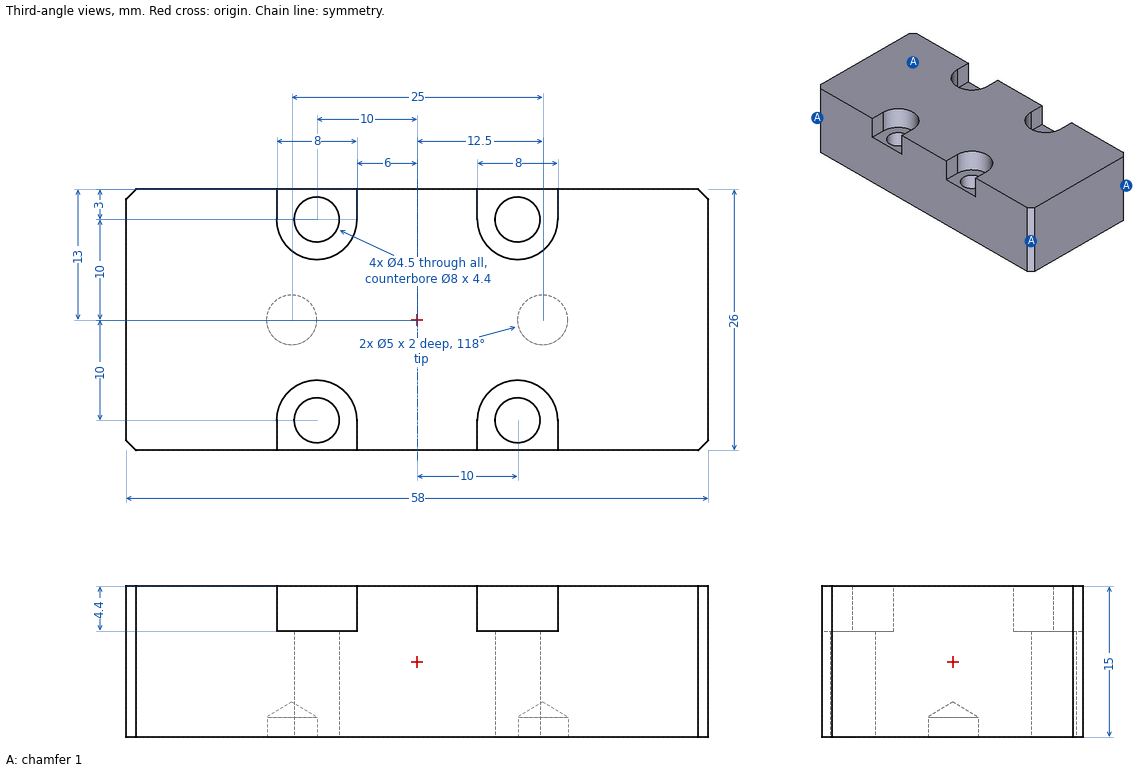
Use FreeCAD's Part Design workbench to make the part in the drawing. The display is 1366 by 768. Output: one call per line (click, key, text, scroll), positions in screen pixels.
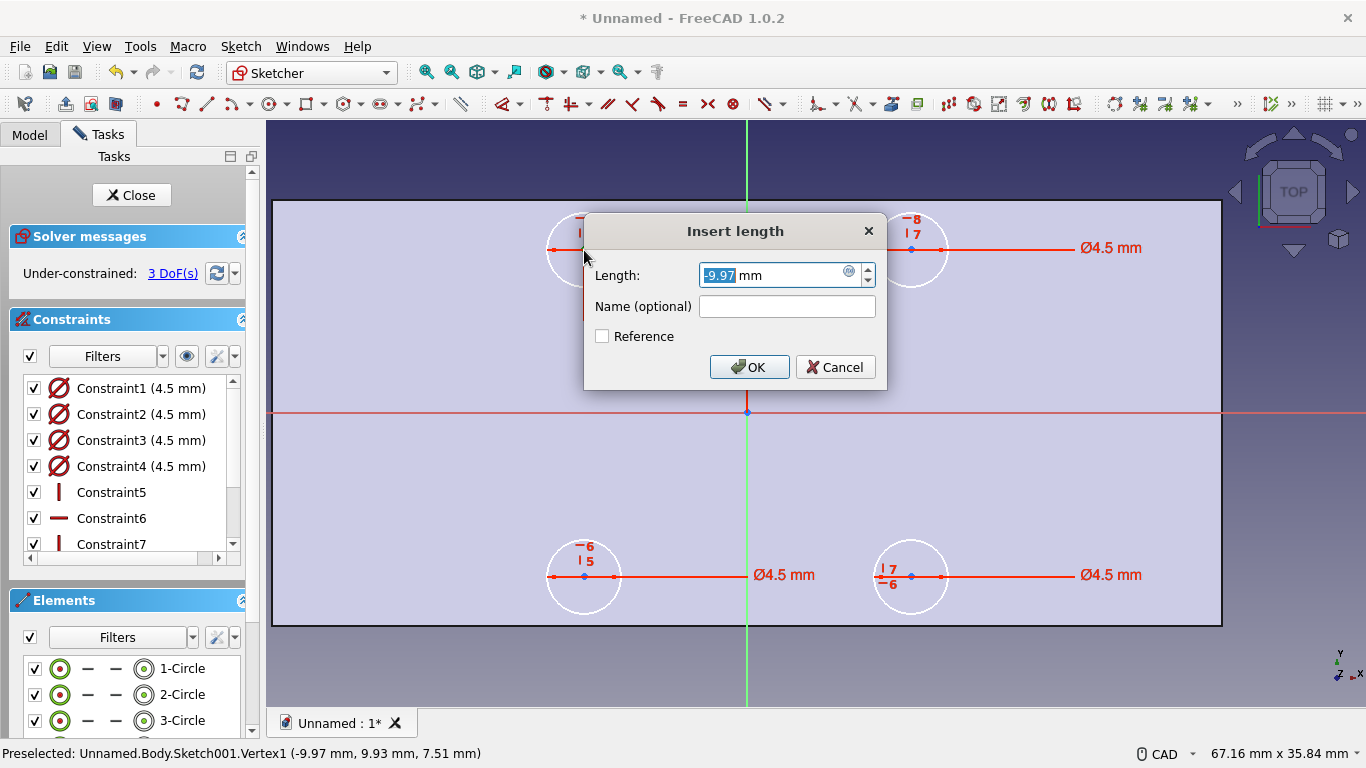
text(-10)
key(Return)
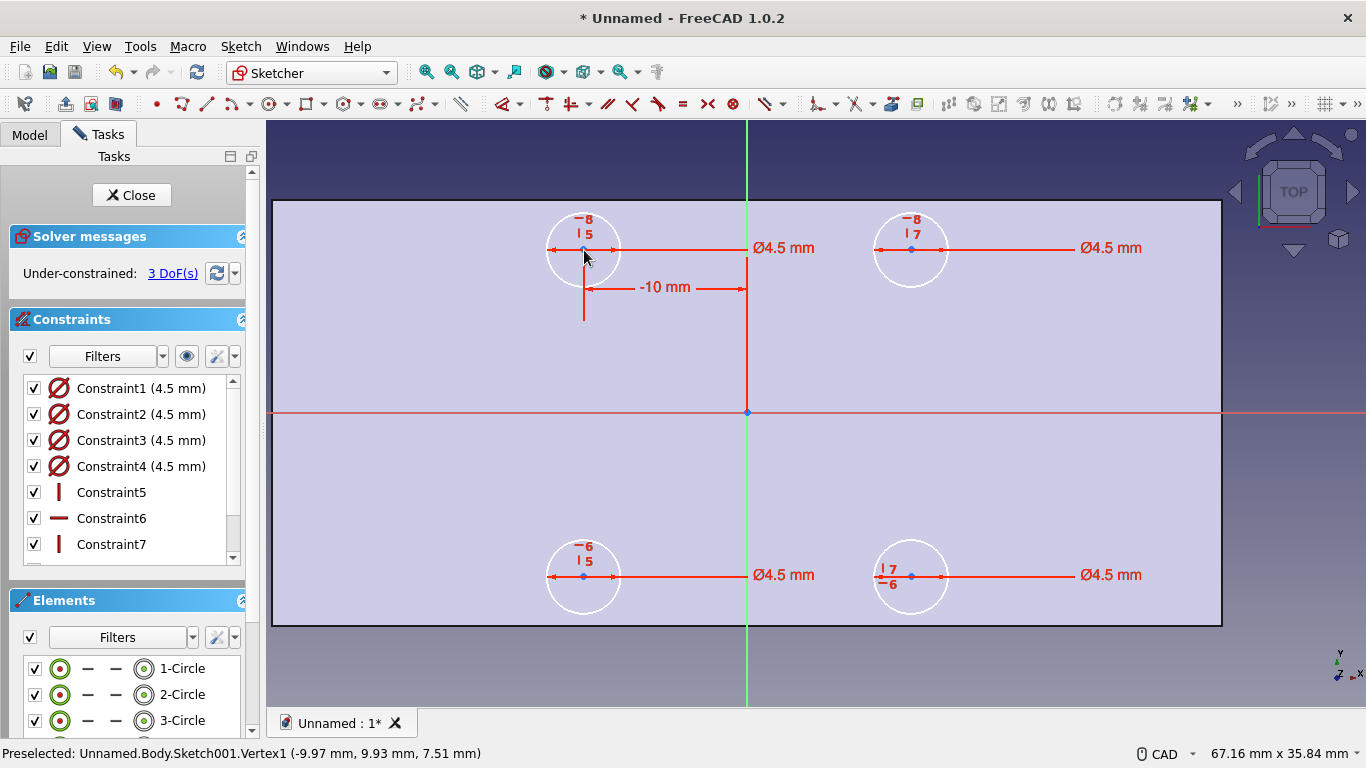
click(584, 250)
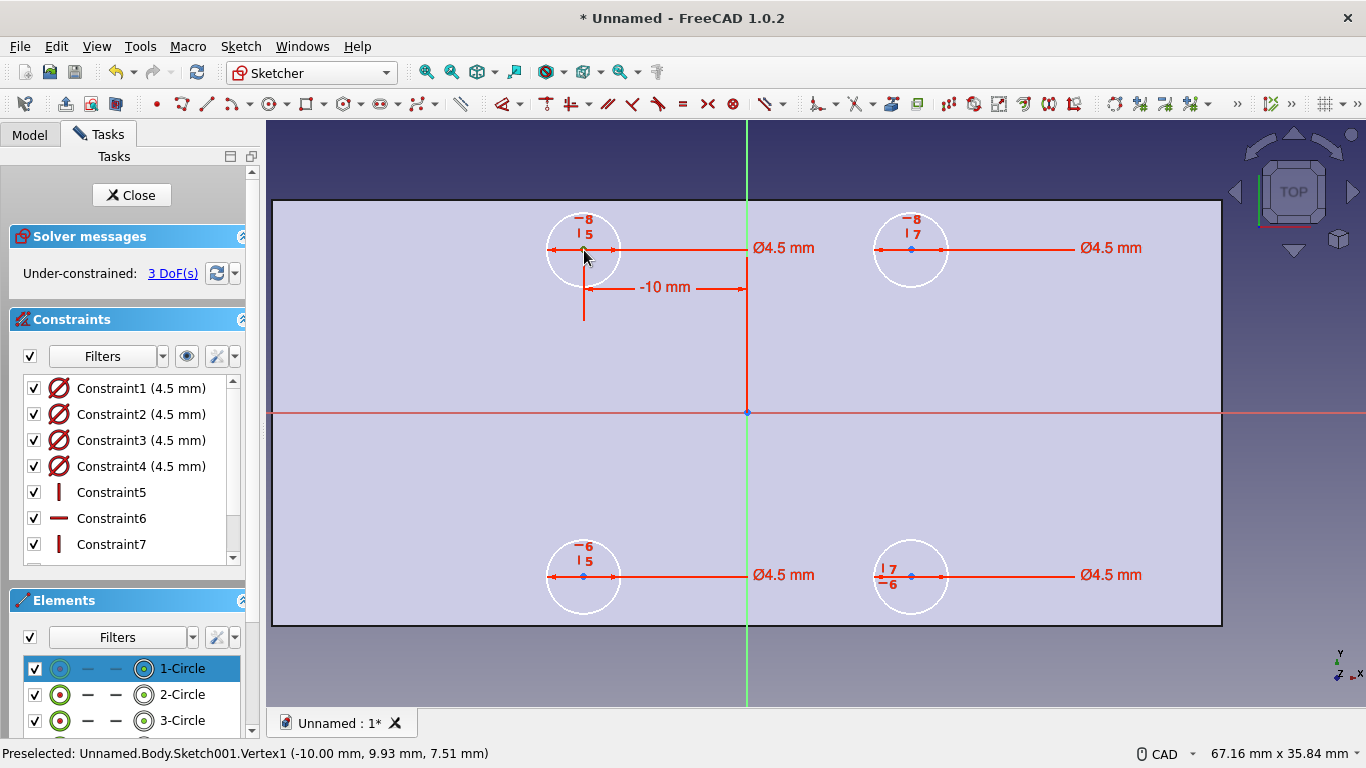
key(i)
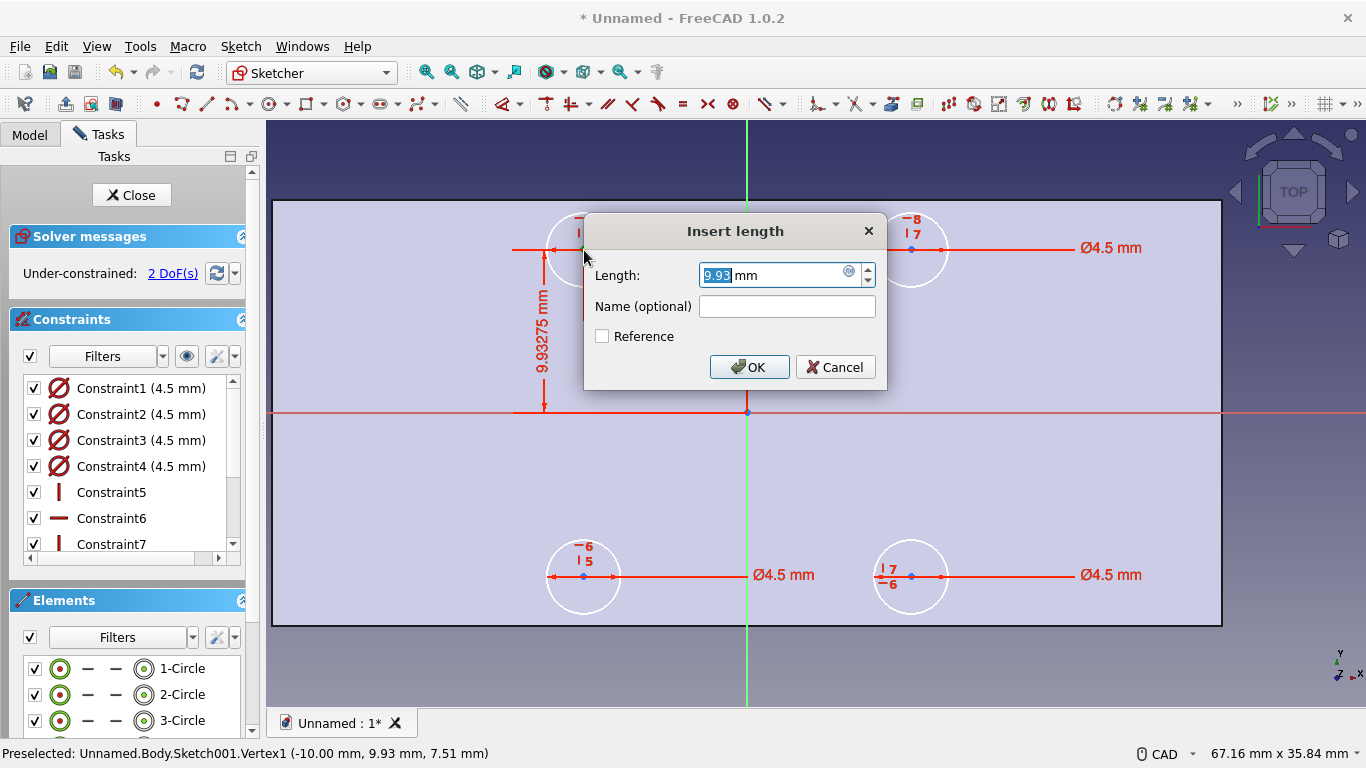
text(10)
key(Return)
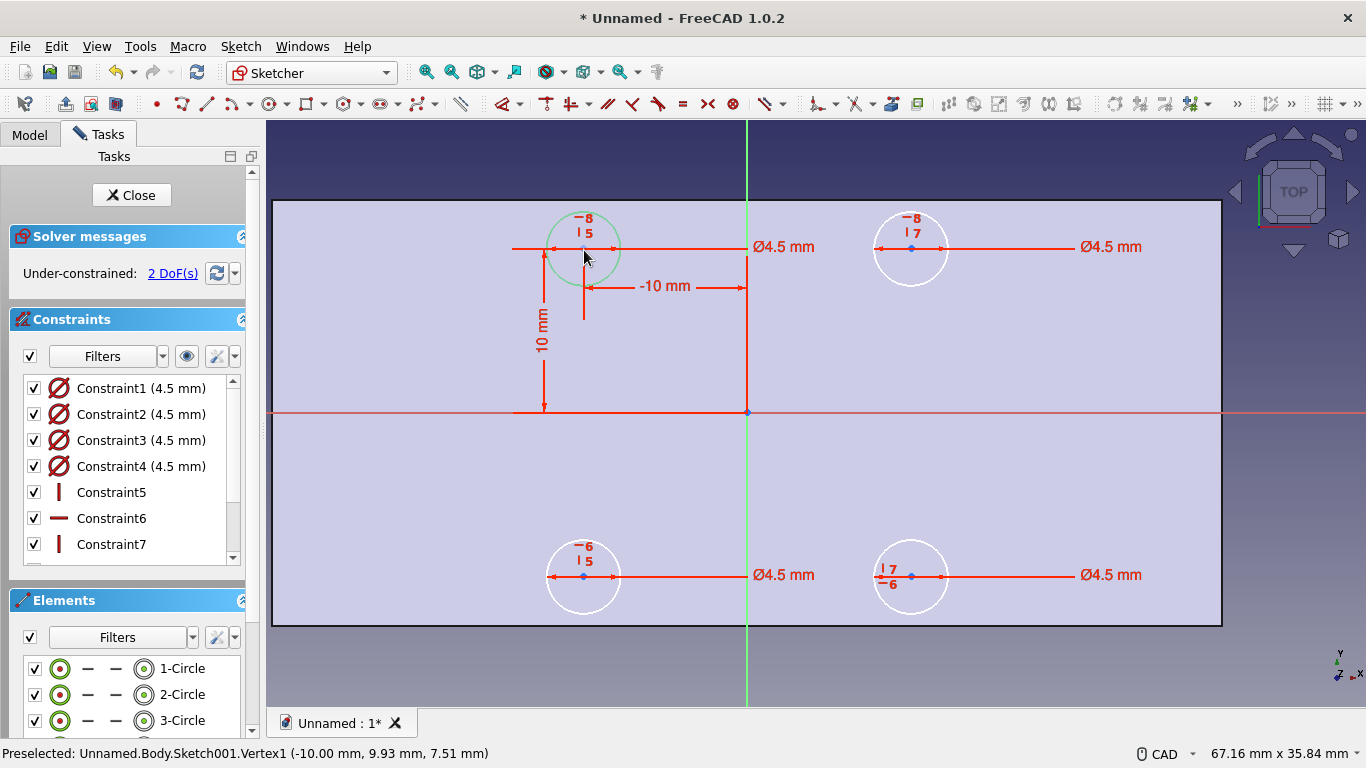
click(584, 577)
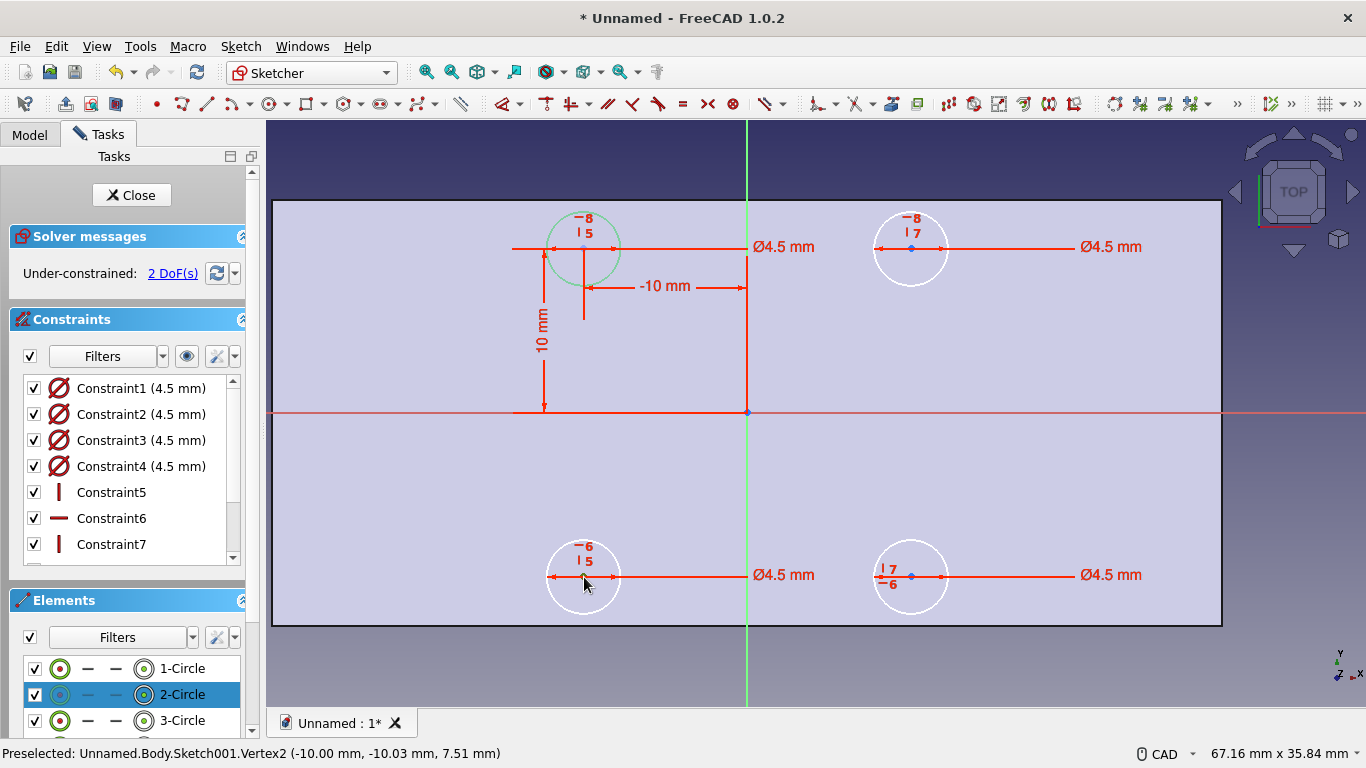
key(i)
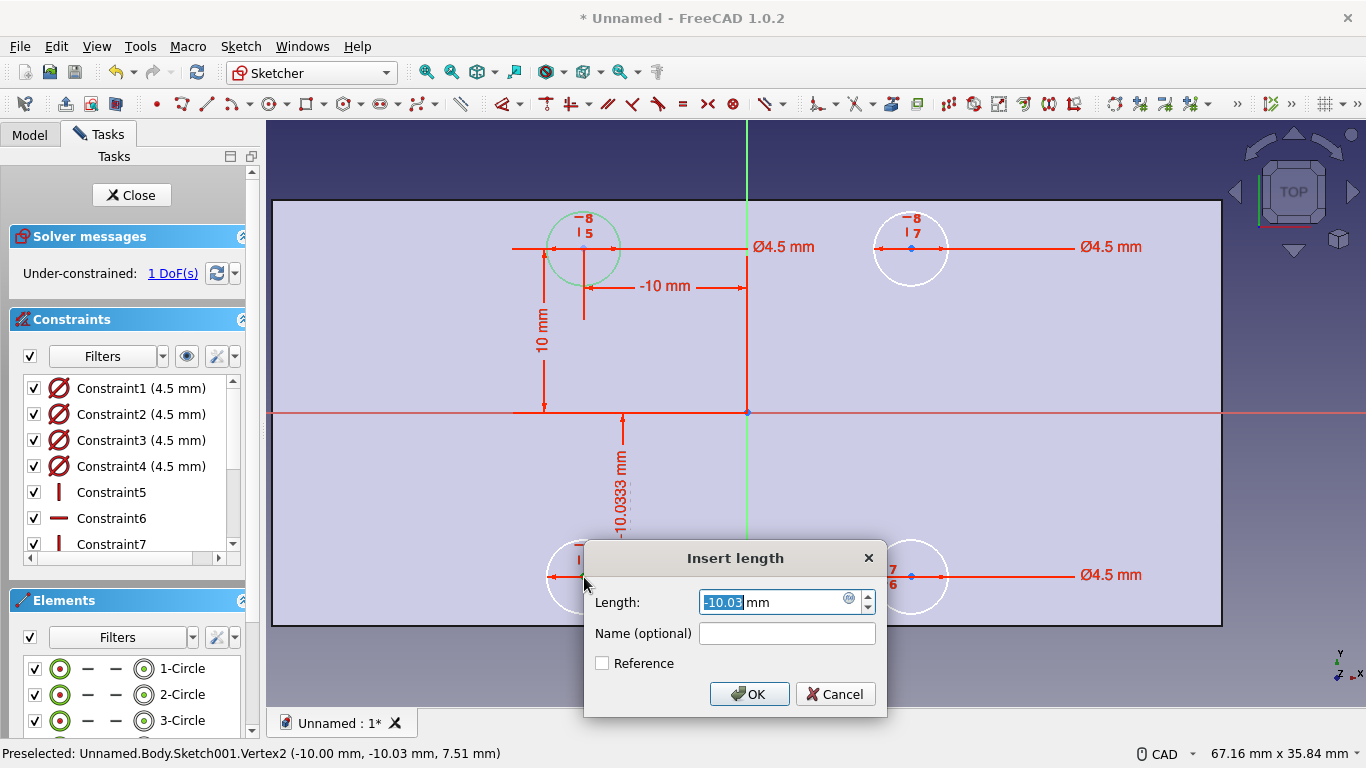
text(-10)
key(Return)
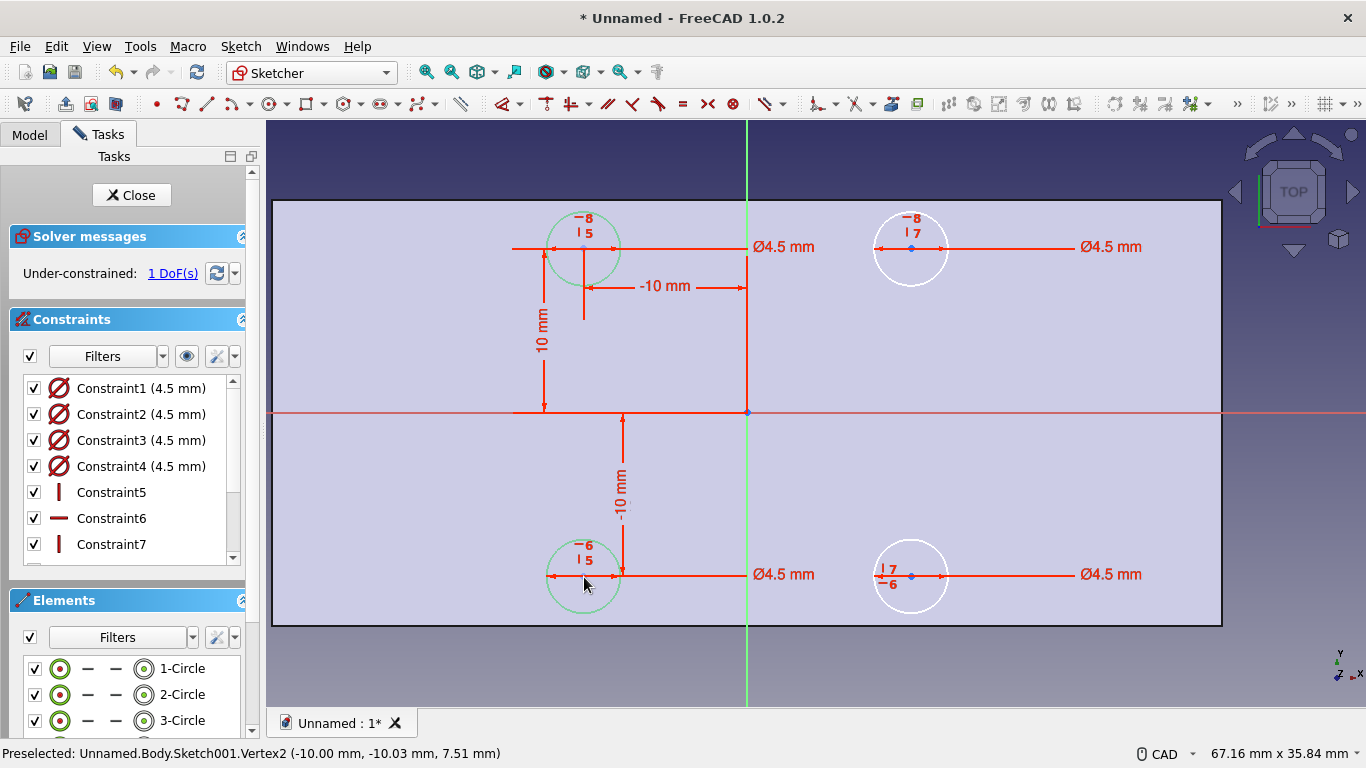
click(911, 576)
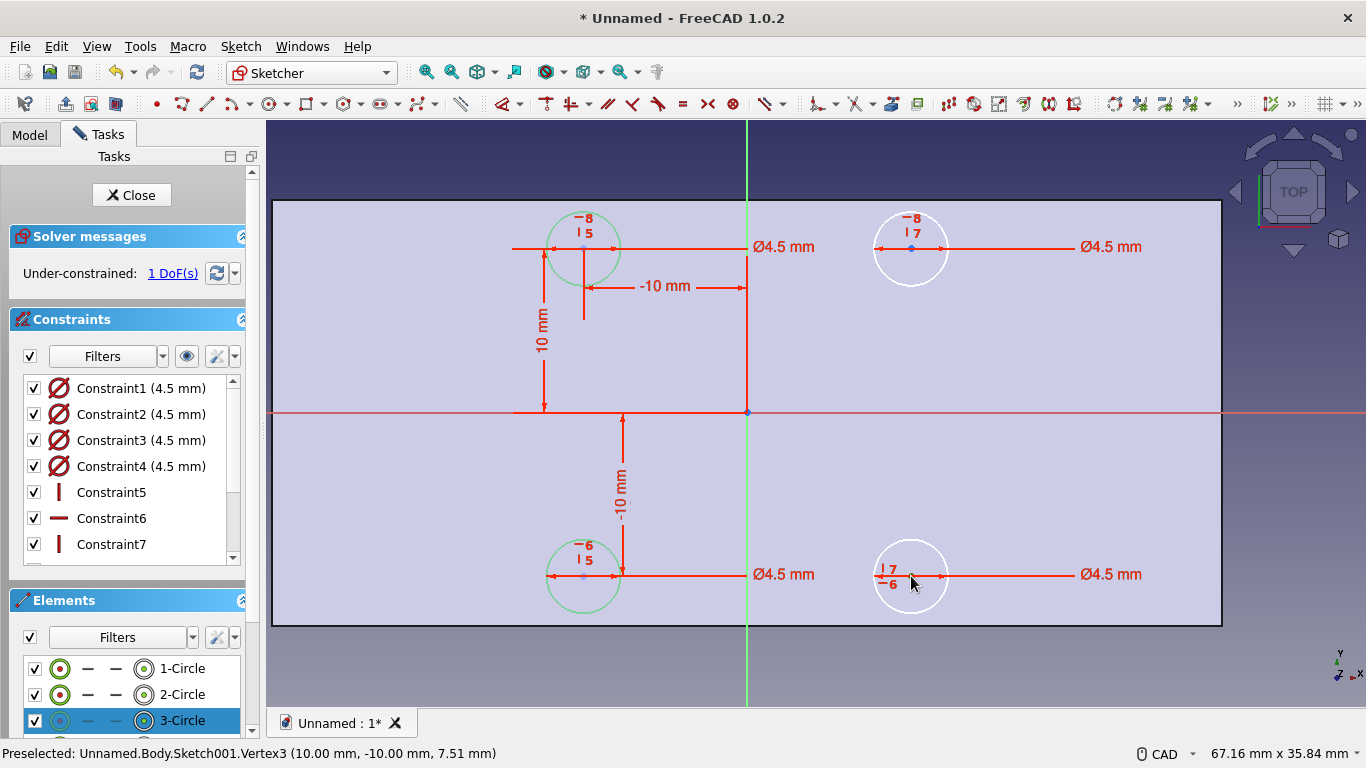
click(520, 104)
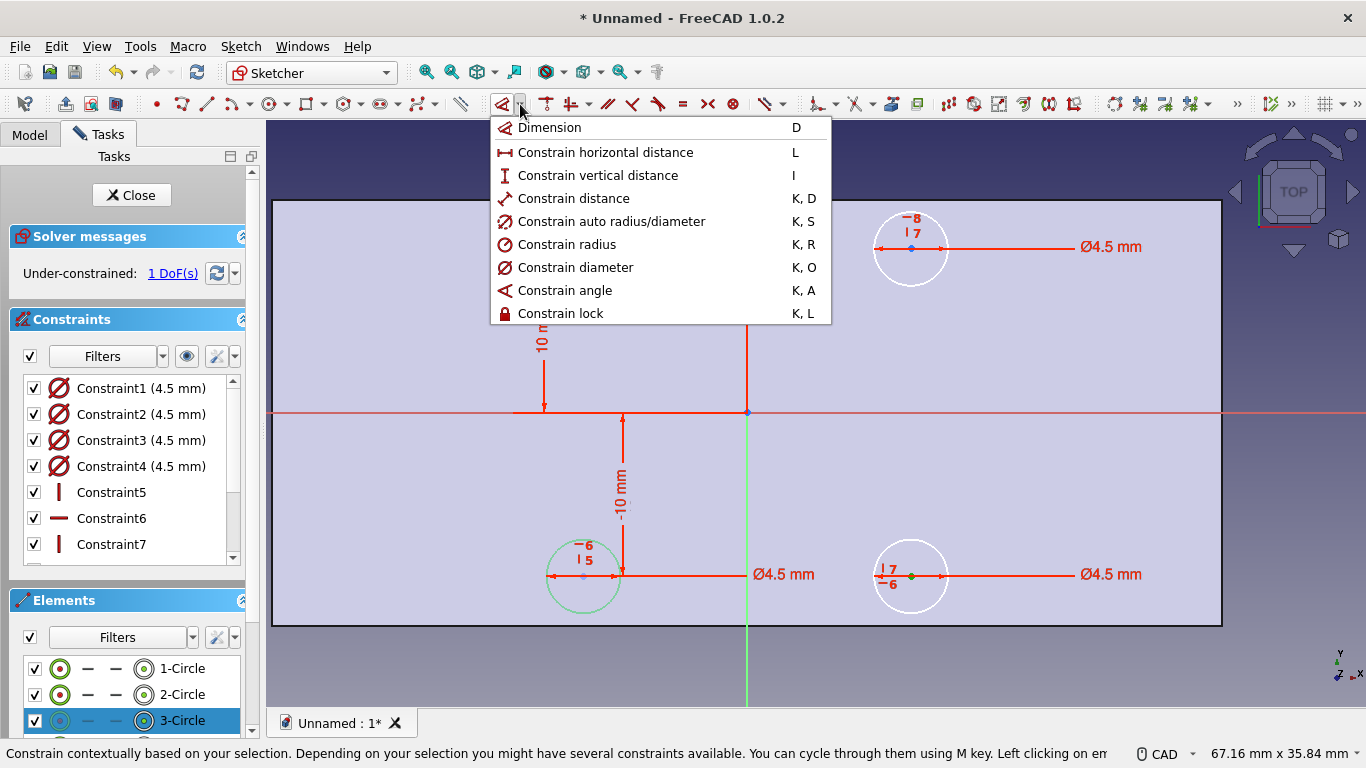
click(661, 152)